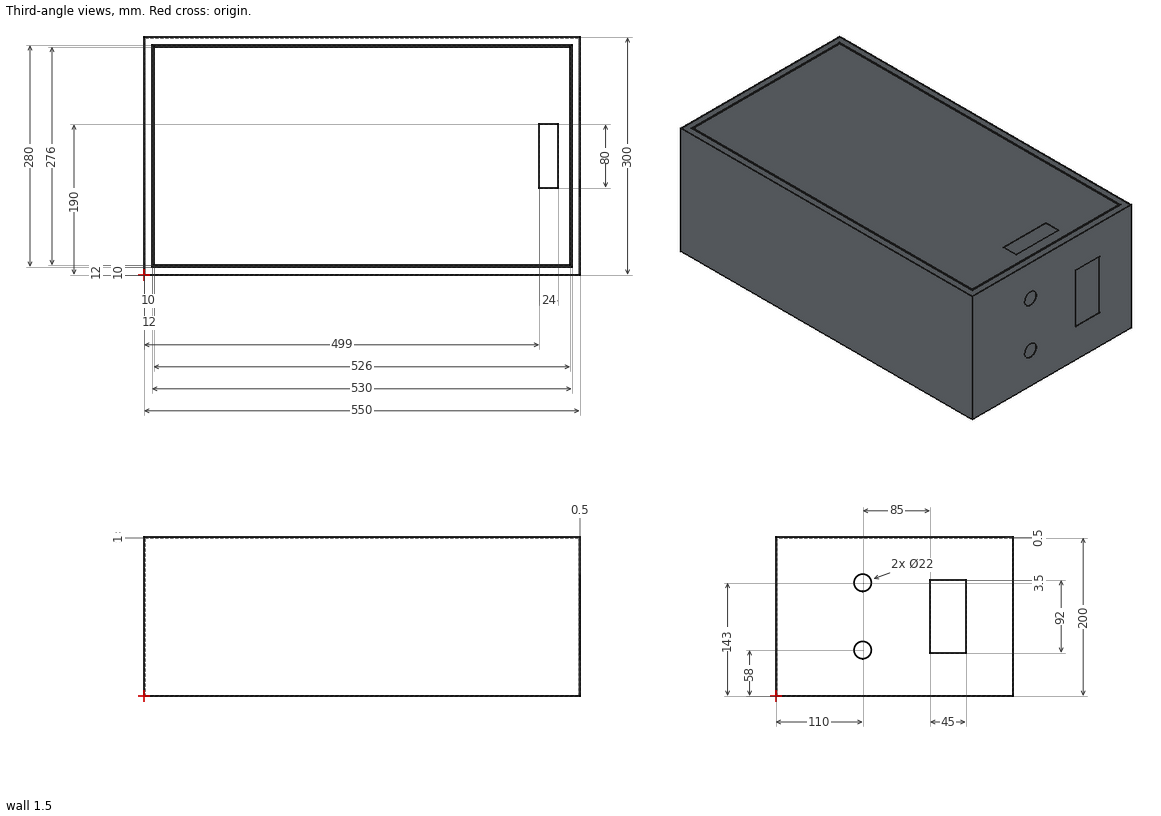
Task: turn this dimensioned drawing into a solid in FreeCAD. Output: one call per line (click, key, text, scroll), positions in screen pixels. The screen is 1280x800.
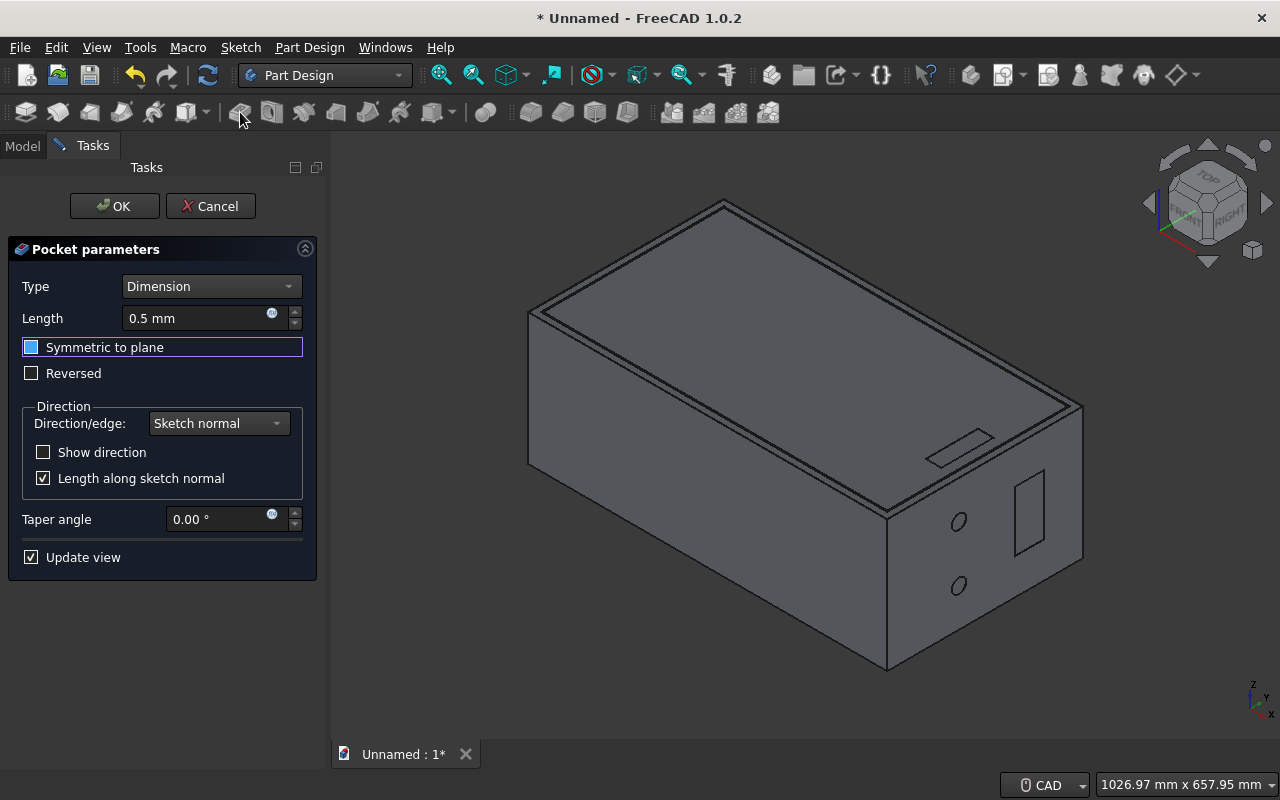
click(115, 206)